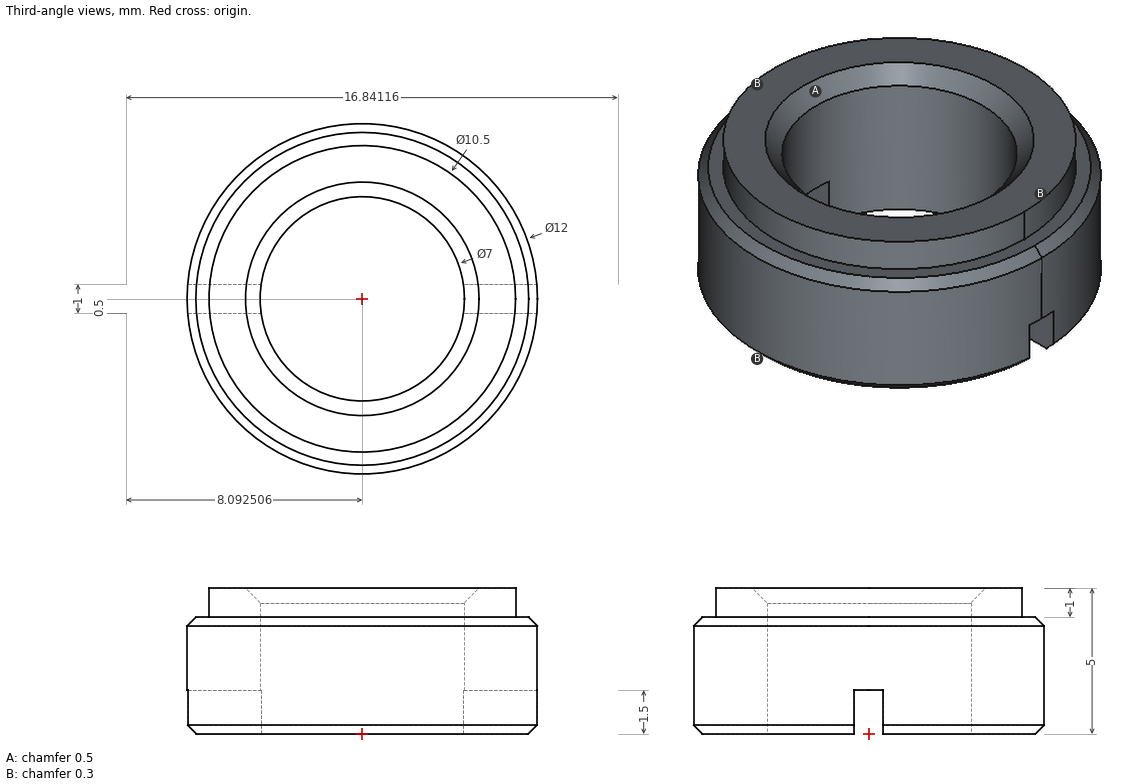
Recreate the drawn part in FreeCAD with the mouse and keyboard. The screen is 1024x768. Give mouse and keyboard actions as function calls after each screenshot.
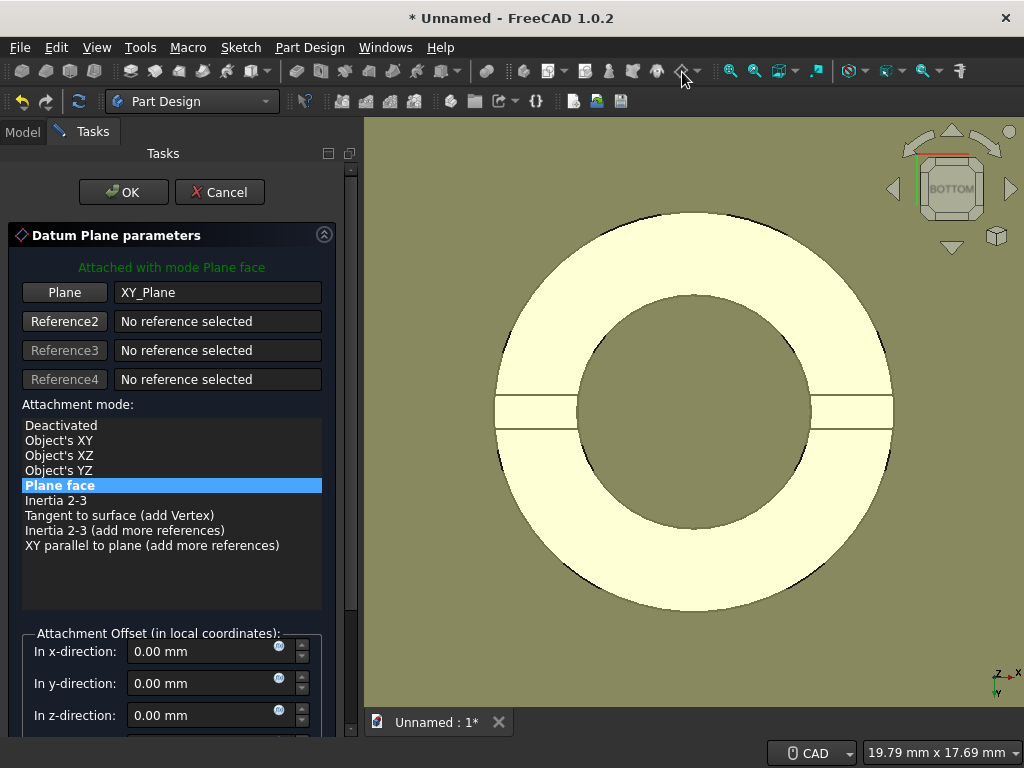
triple_click(210, 715)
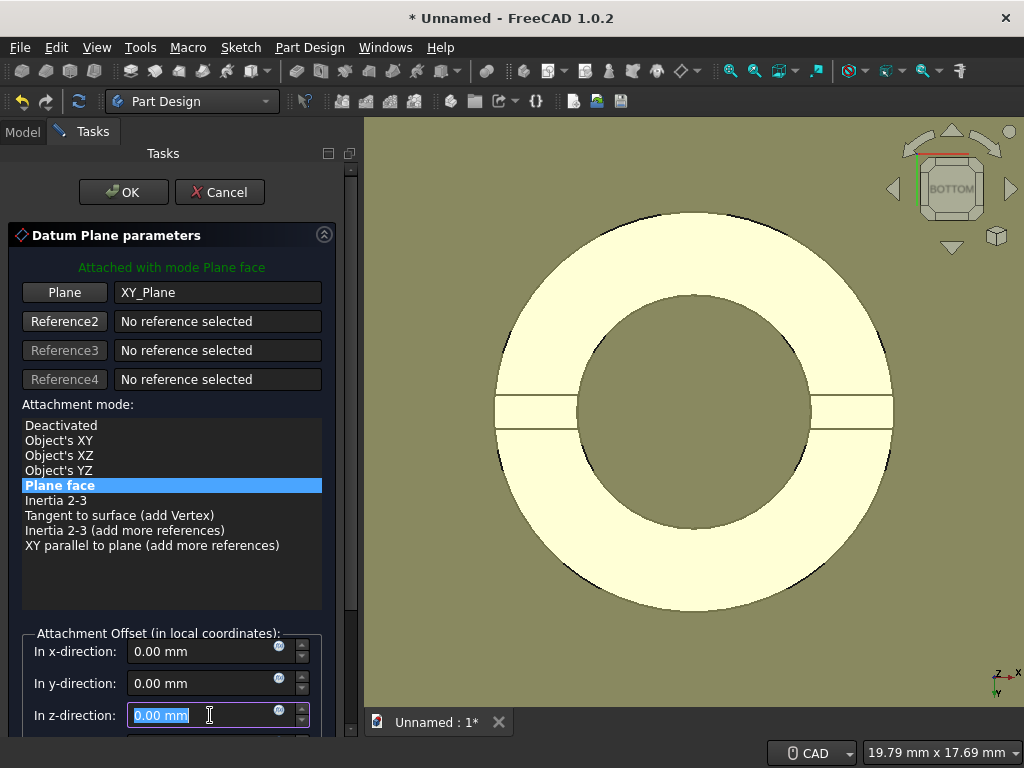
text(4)
key(Tab)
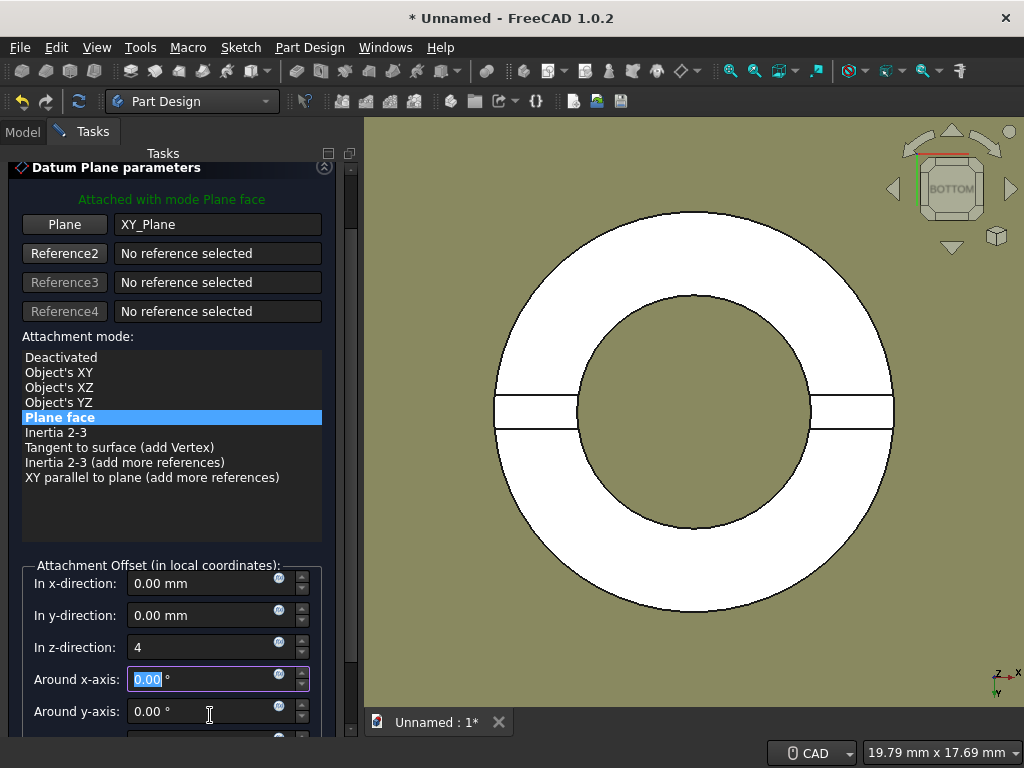
scroll(351, 450, up, 2)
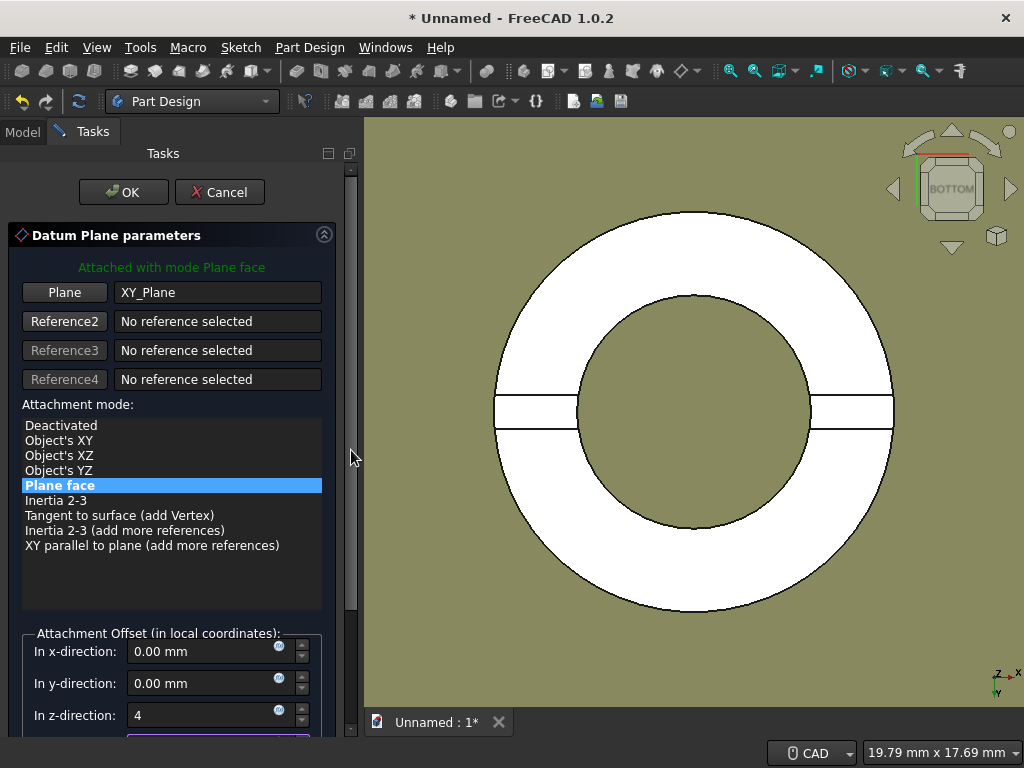
click(124, 192)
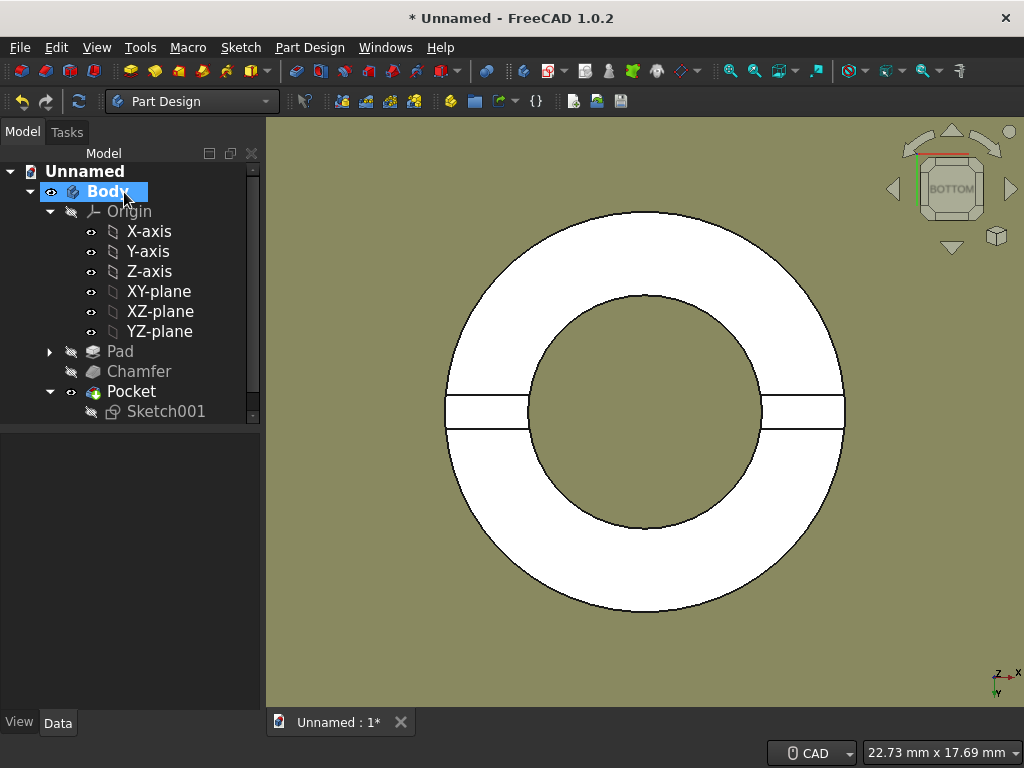
scroll(100, 287, down, 3)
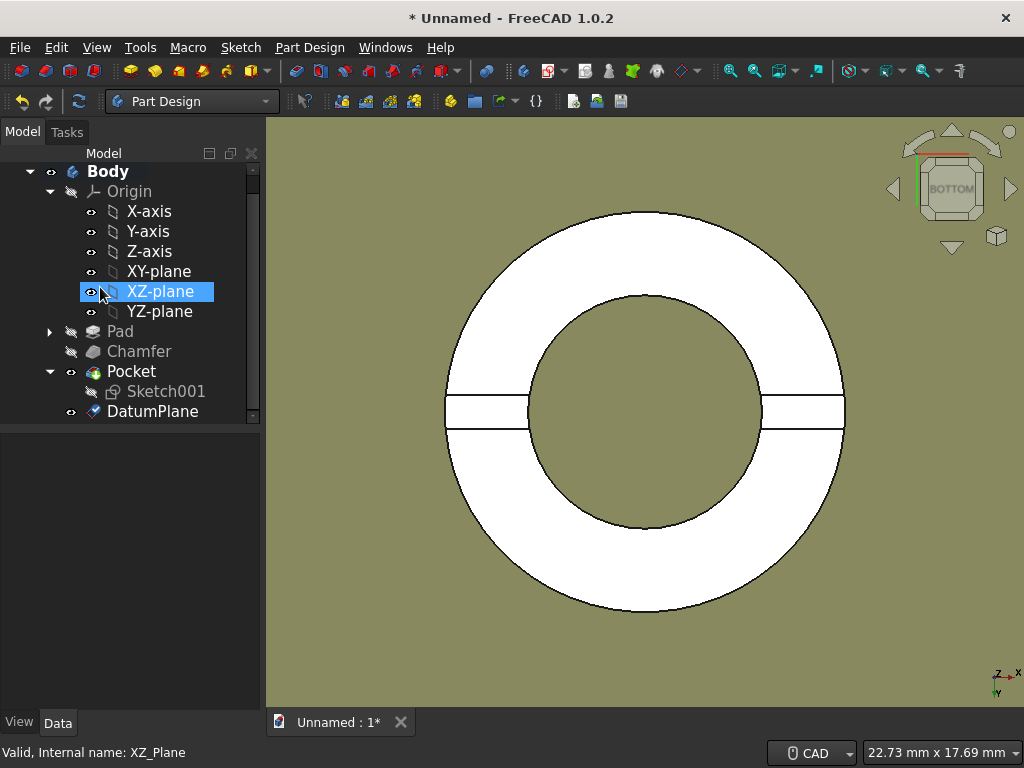
click(116, 412)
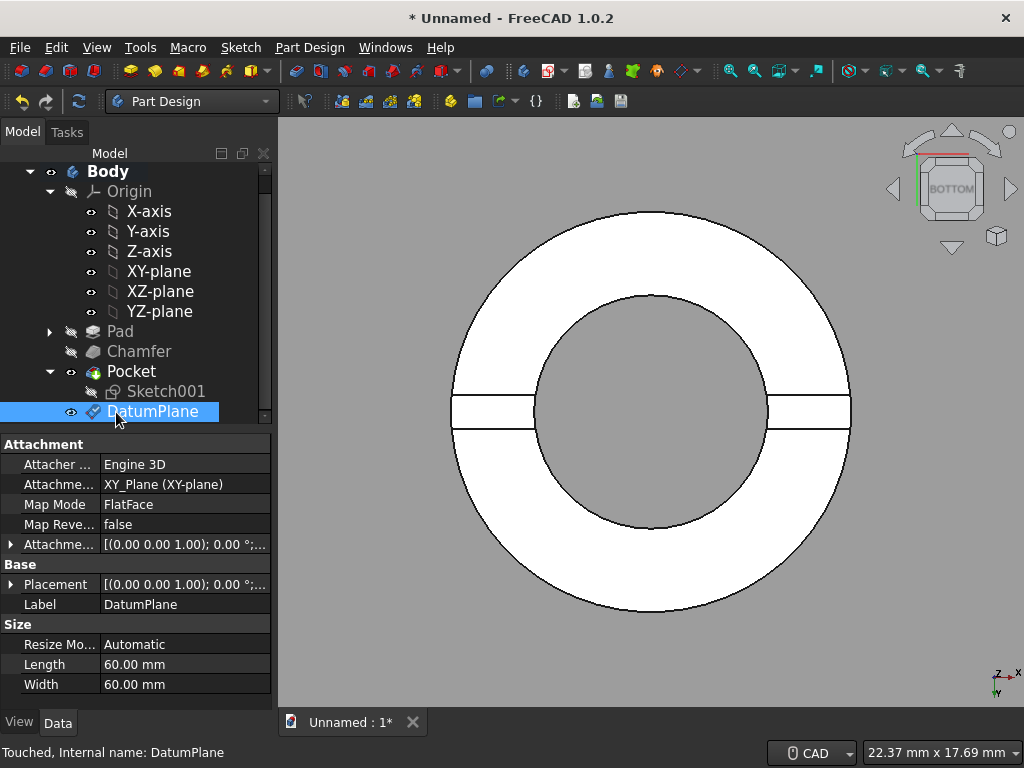
click(548, 72)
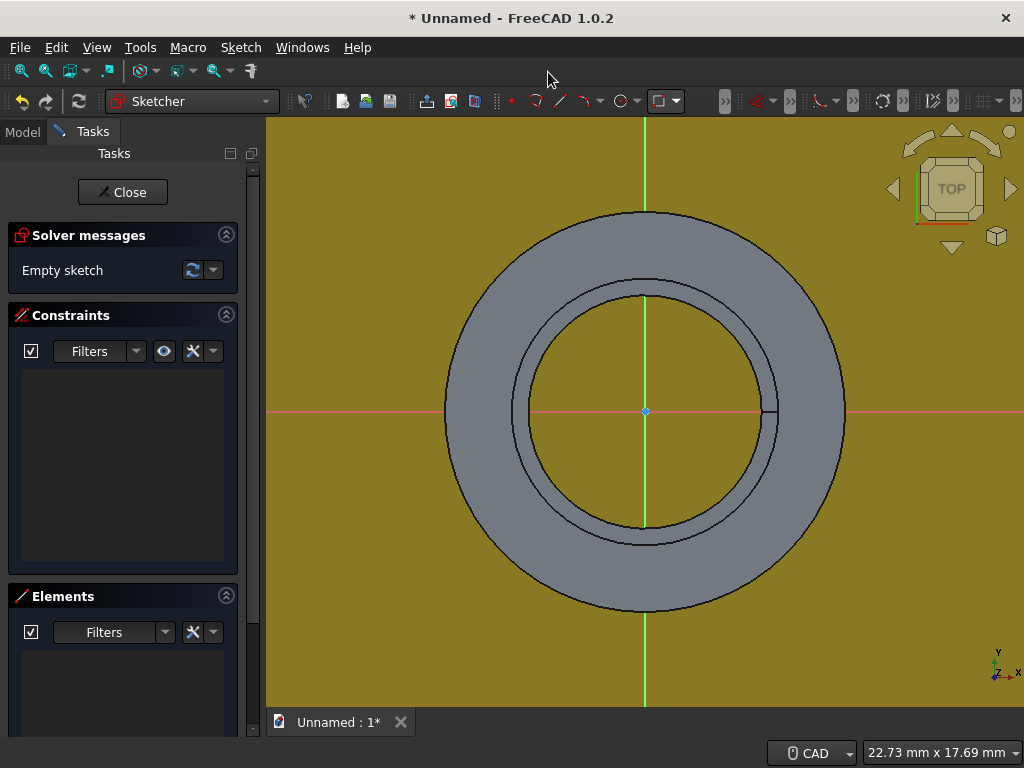
click(476, 102)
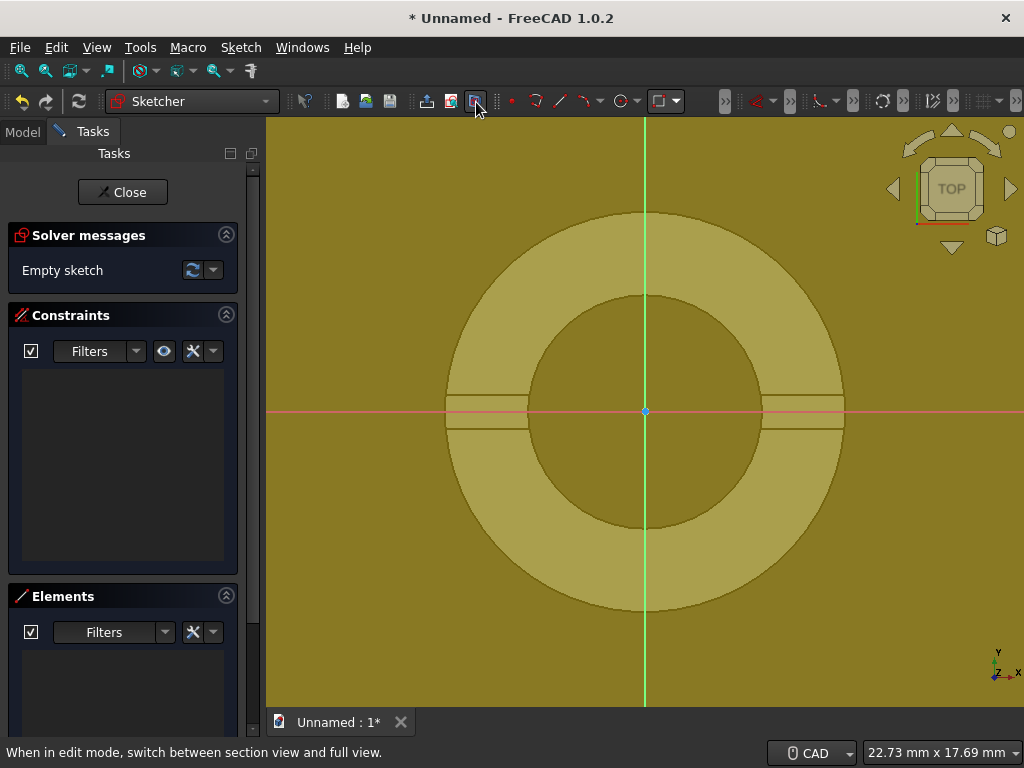
scroll(294, 412, down, 1)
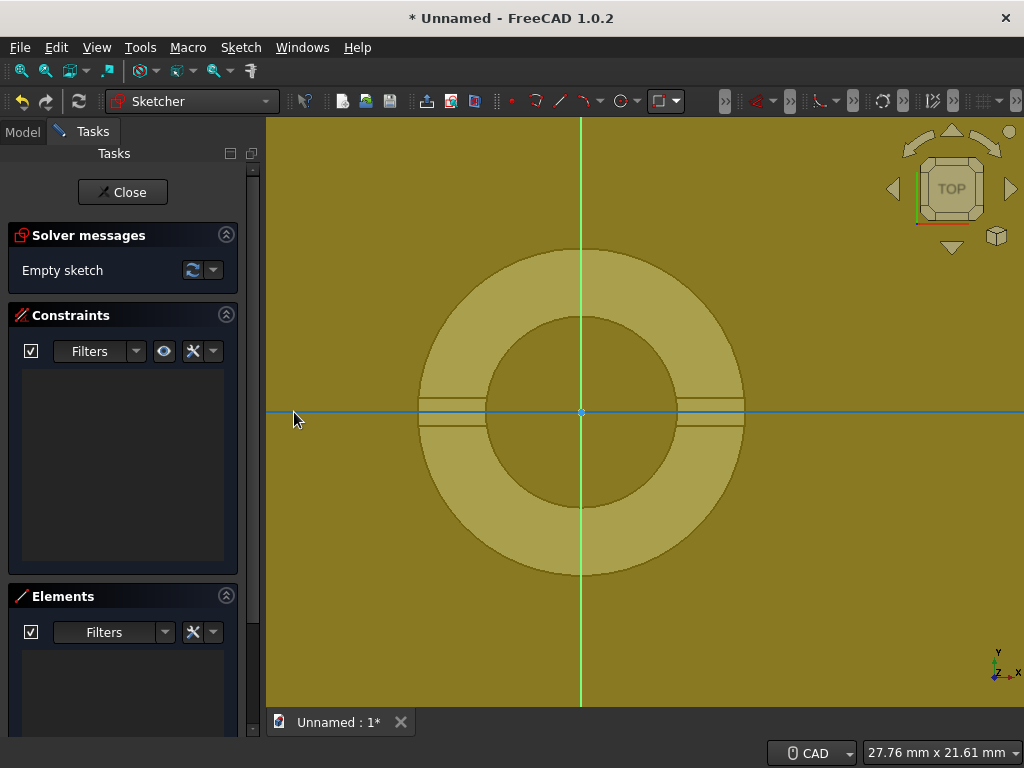
key(g)
key(c)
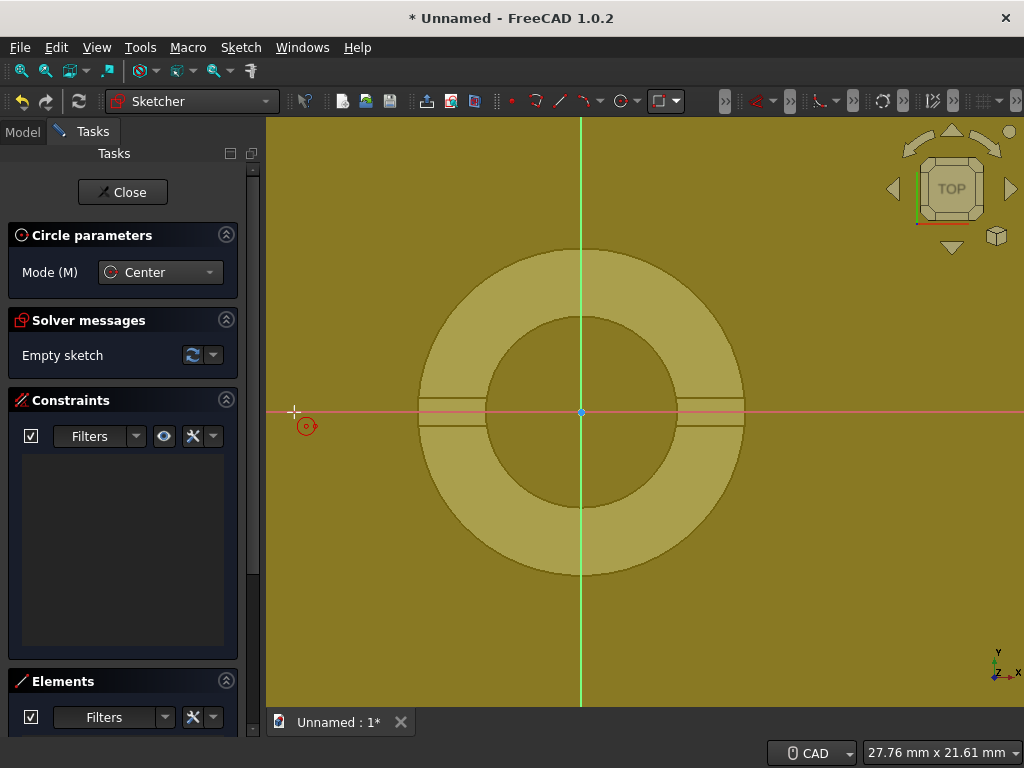
click(581, 412)
move(697, 296)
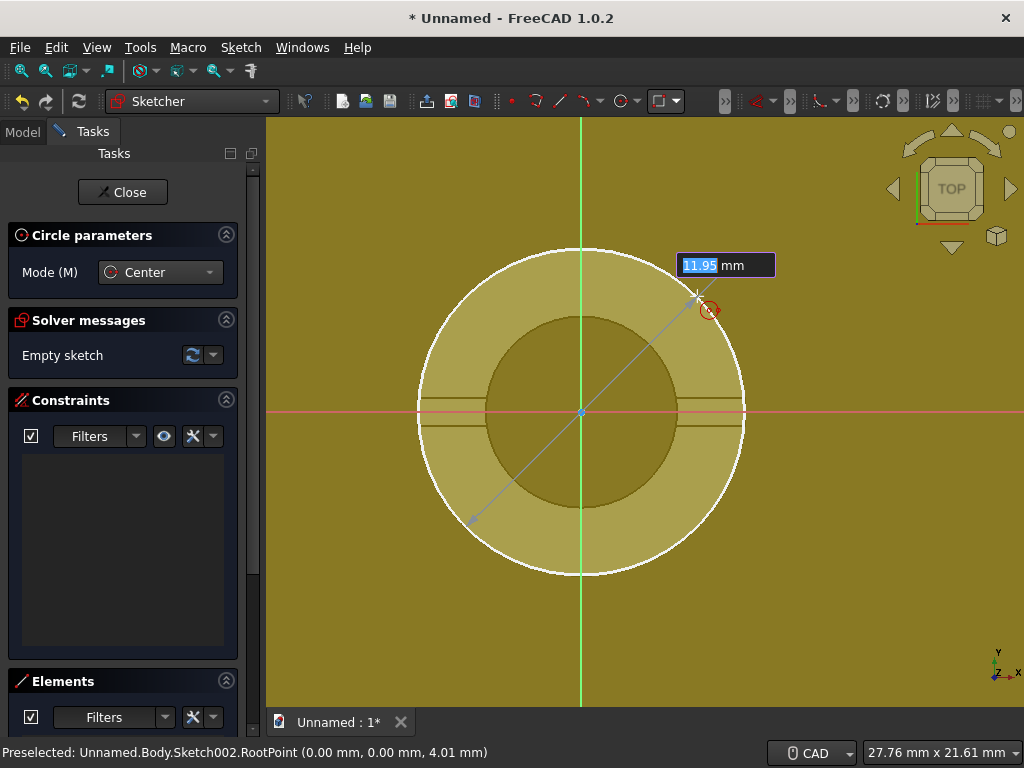
text(12)
key(Return)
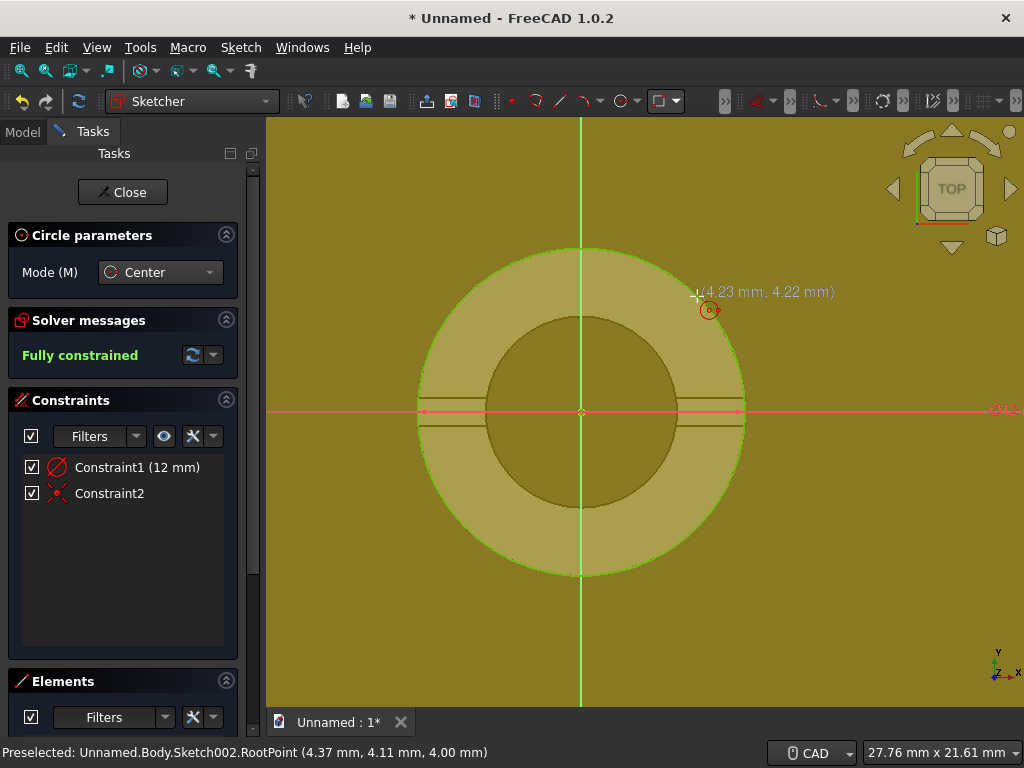
click(581, 412)
move(683, 311)